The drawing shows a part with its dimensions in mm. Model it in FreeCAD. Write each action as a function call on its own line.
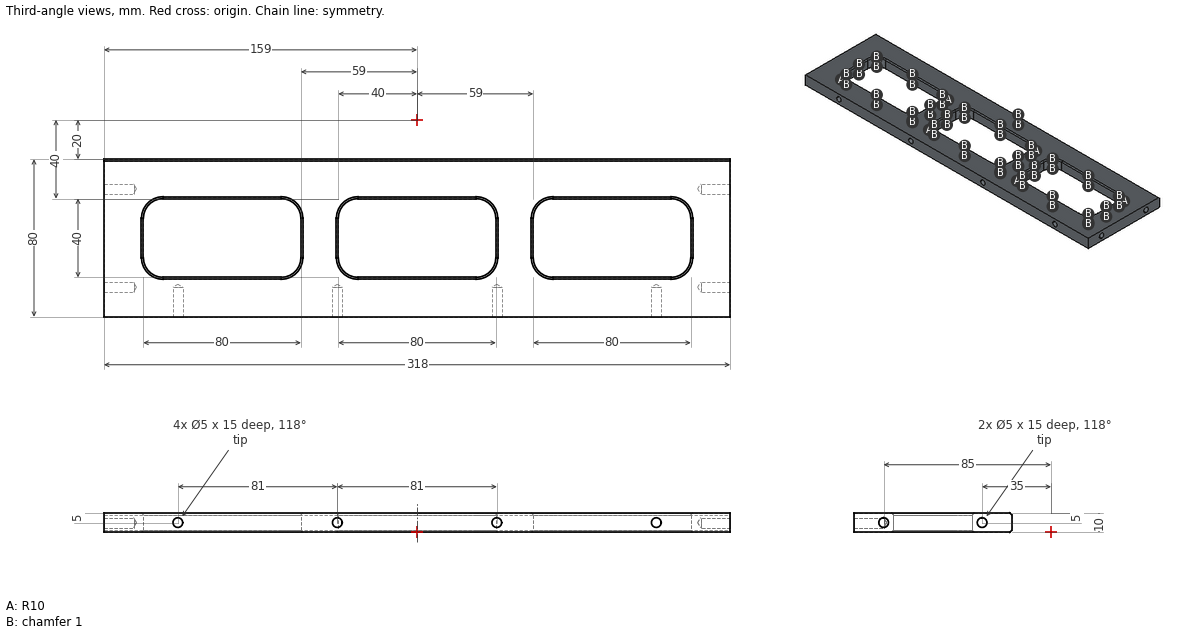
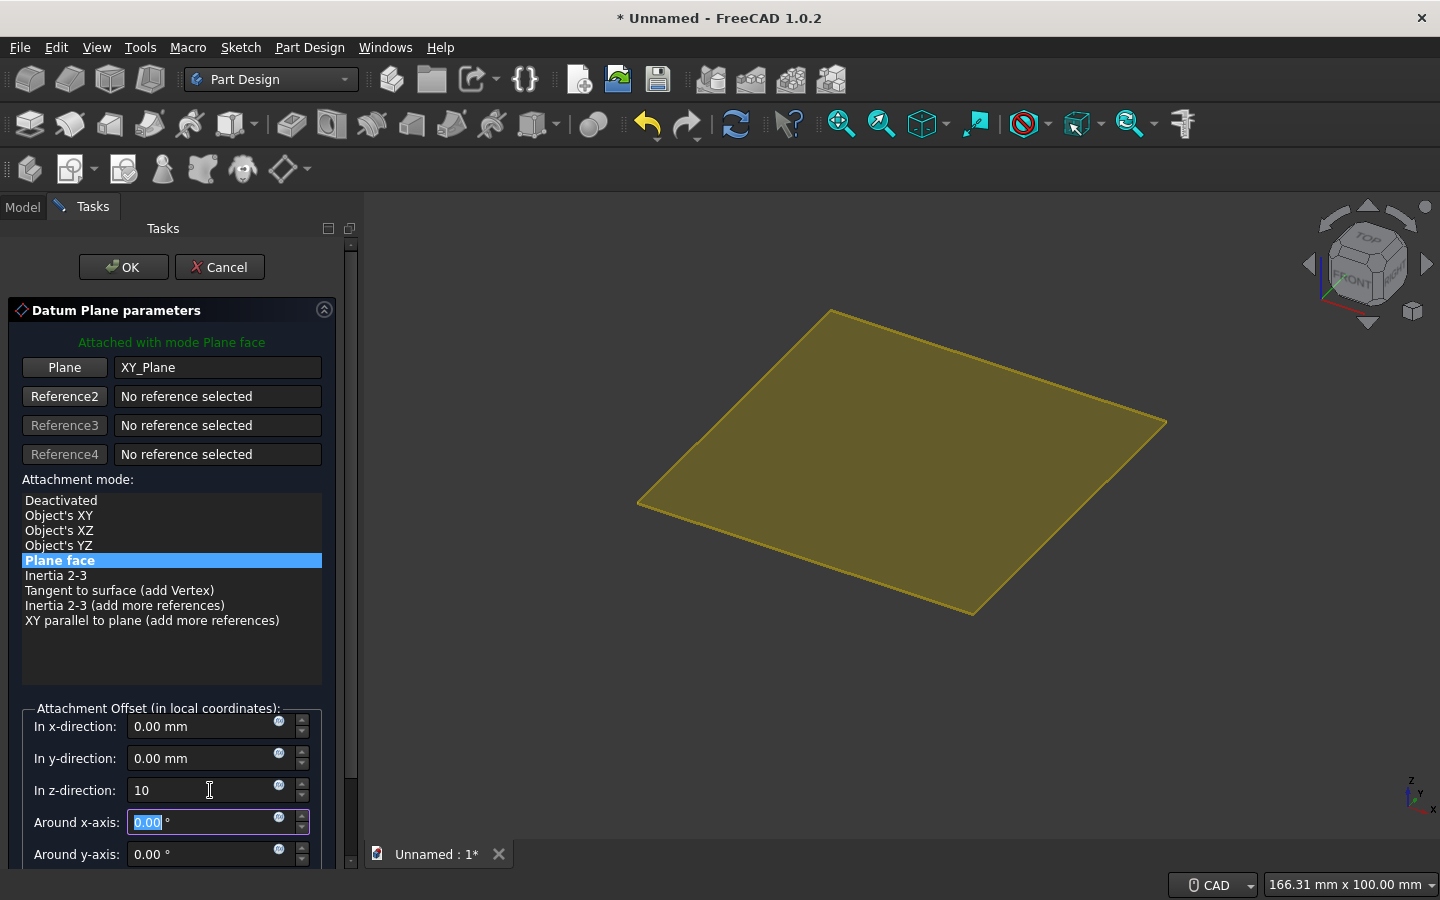
click(124, 267)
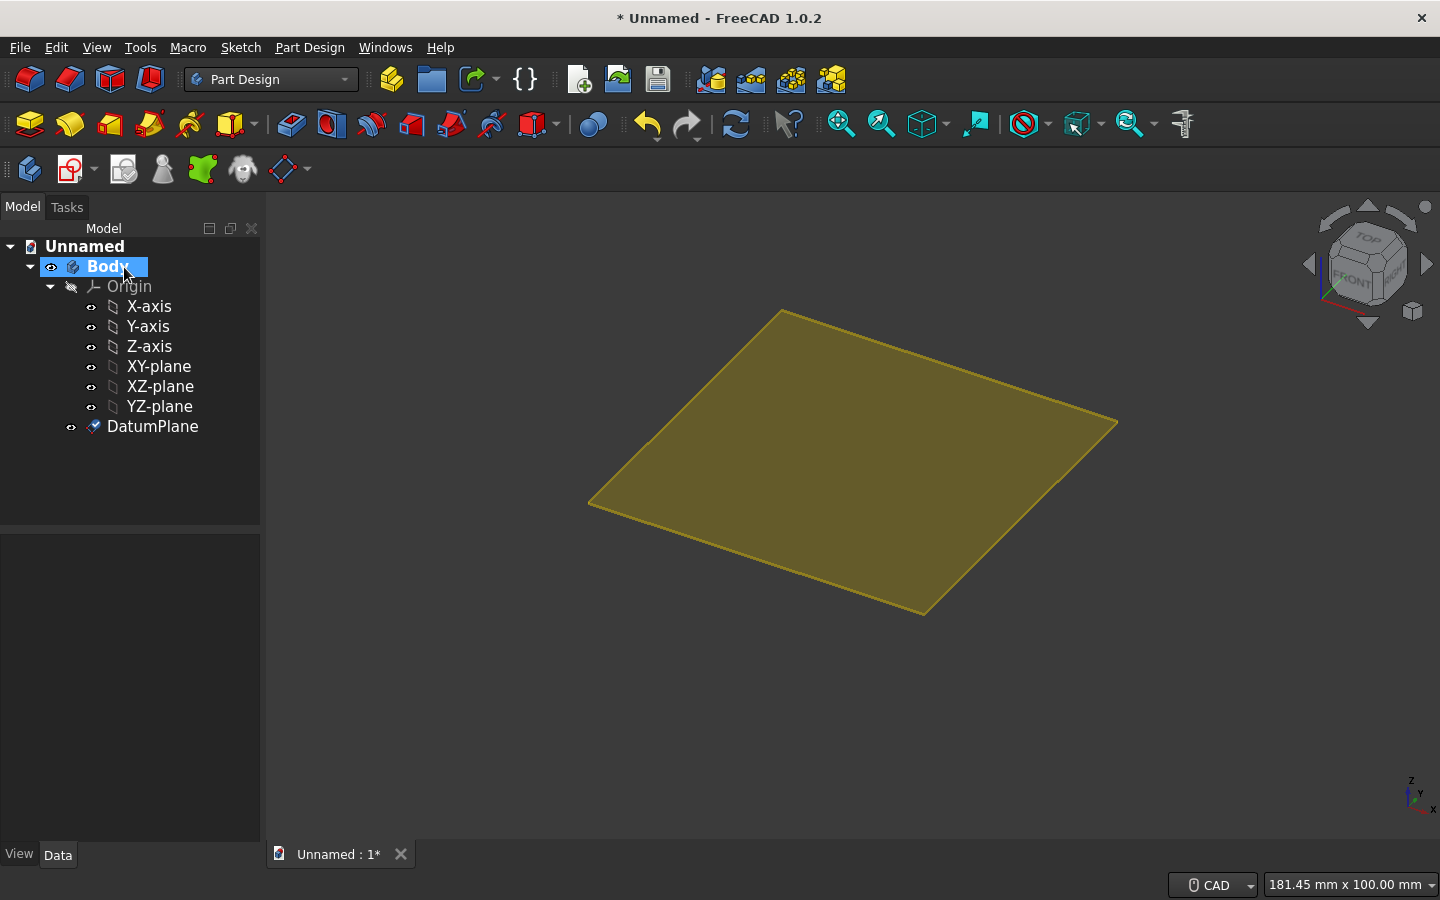
click(116, 427)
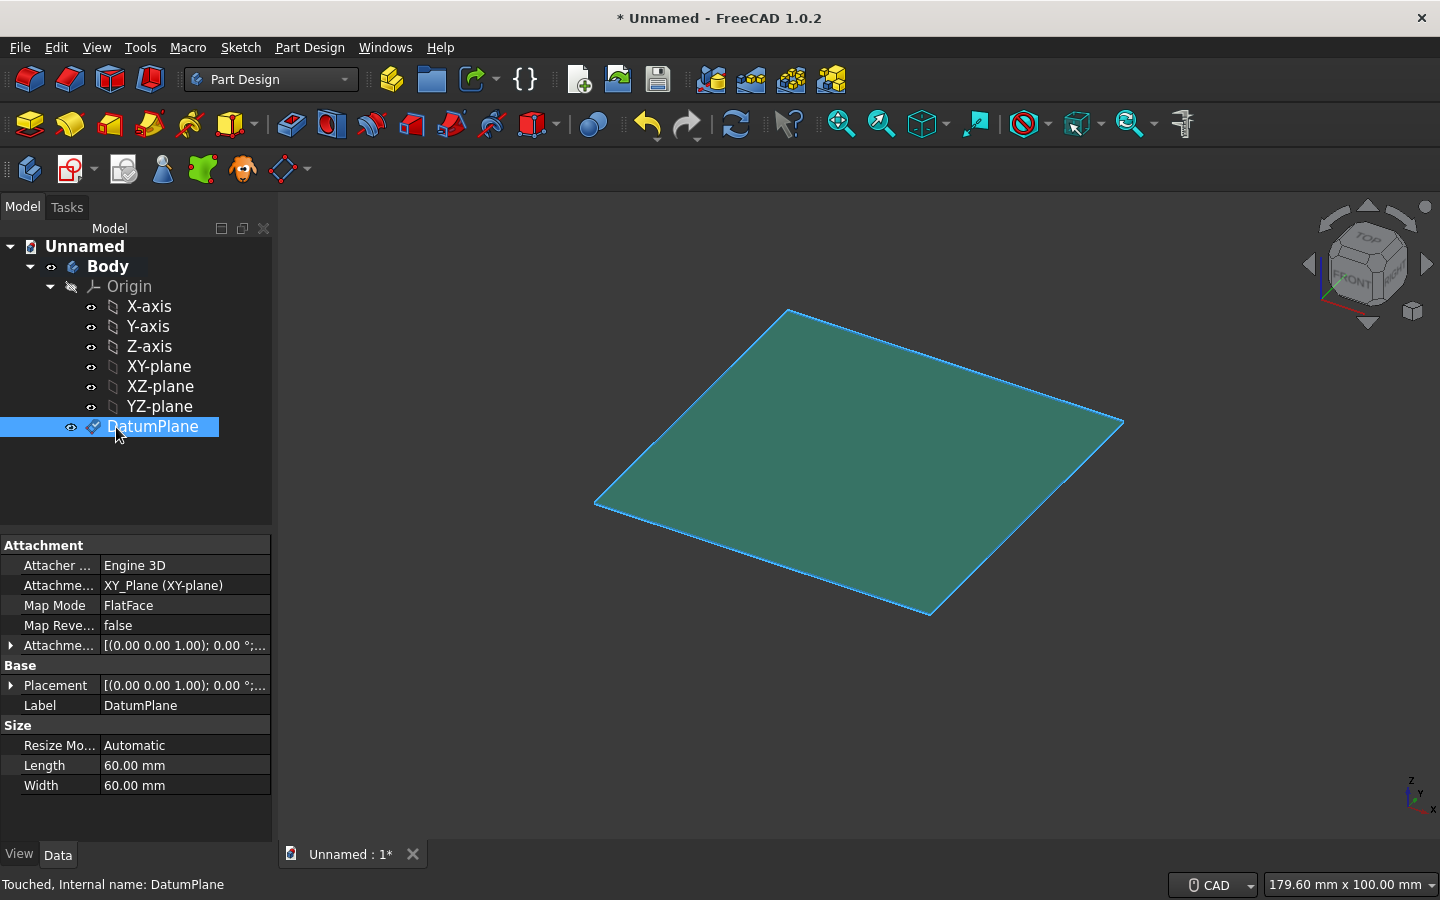
click(70, 170)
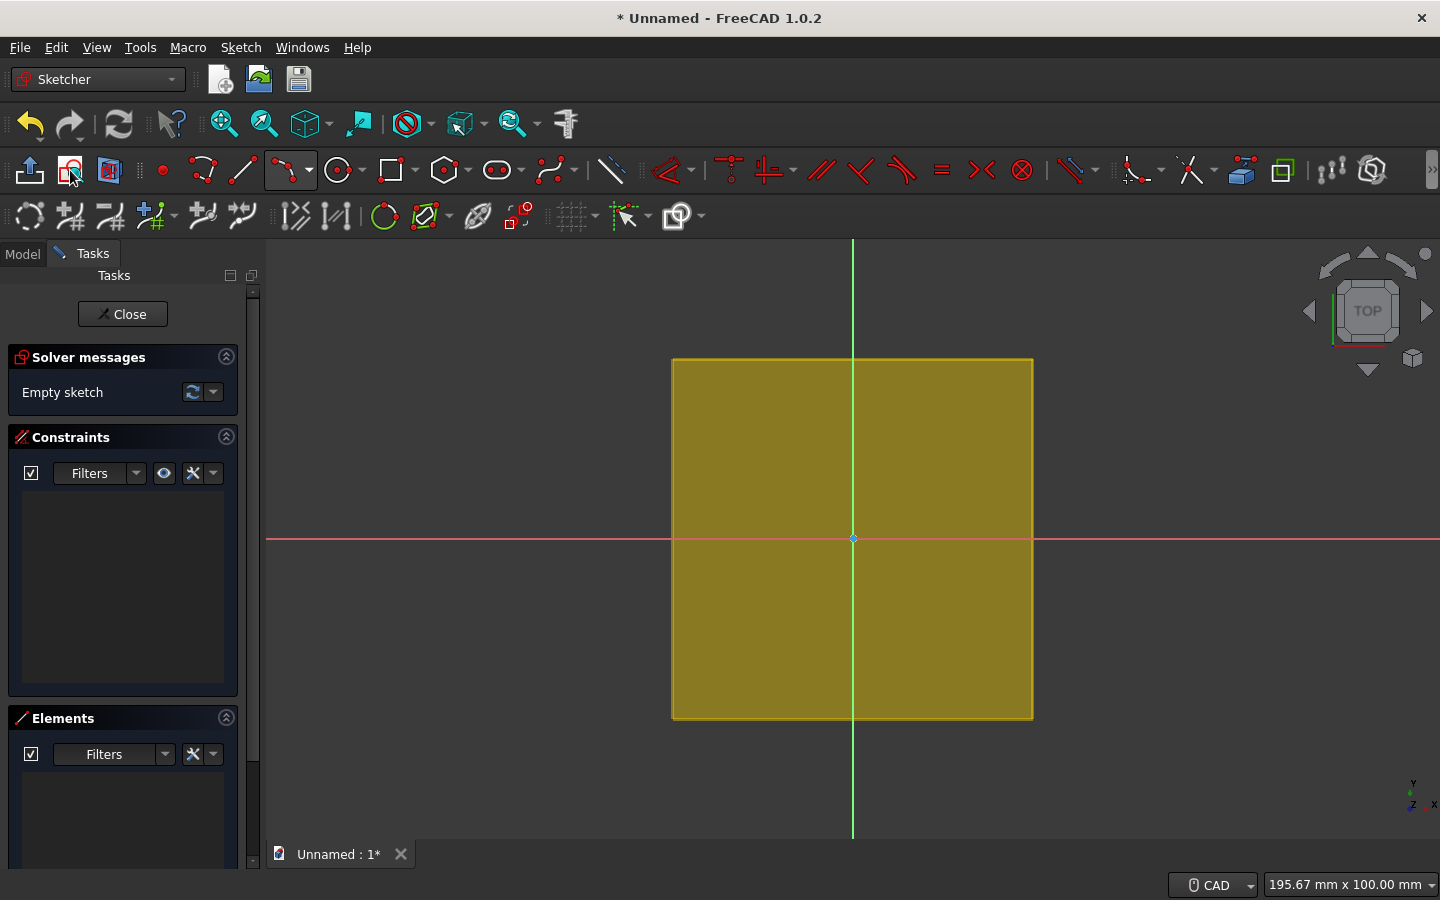
scroll(745, 364, down, 5)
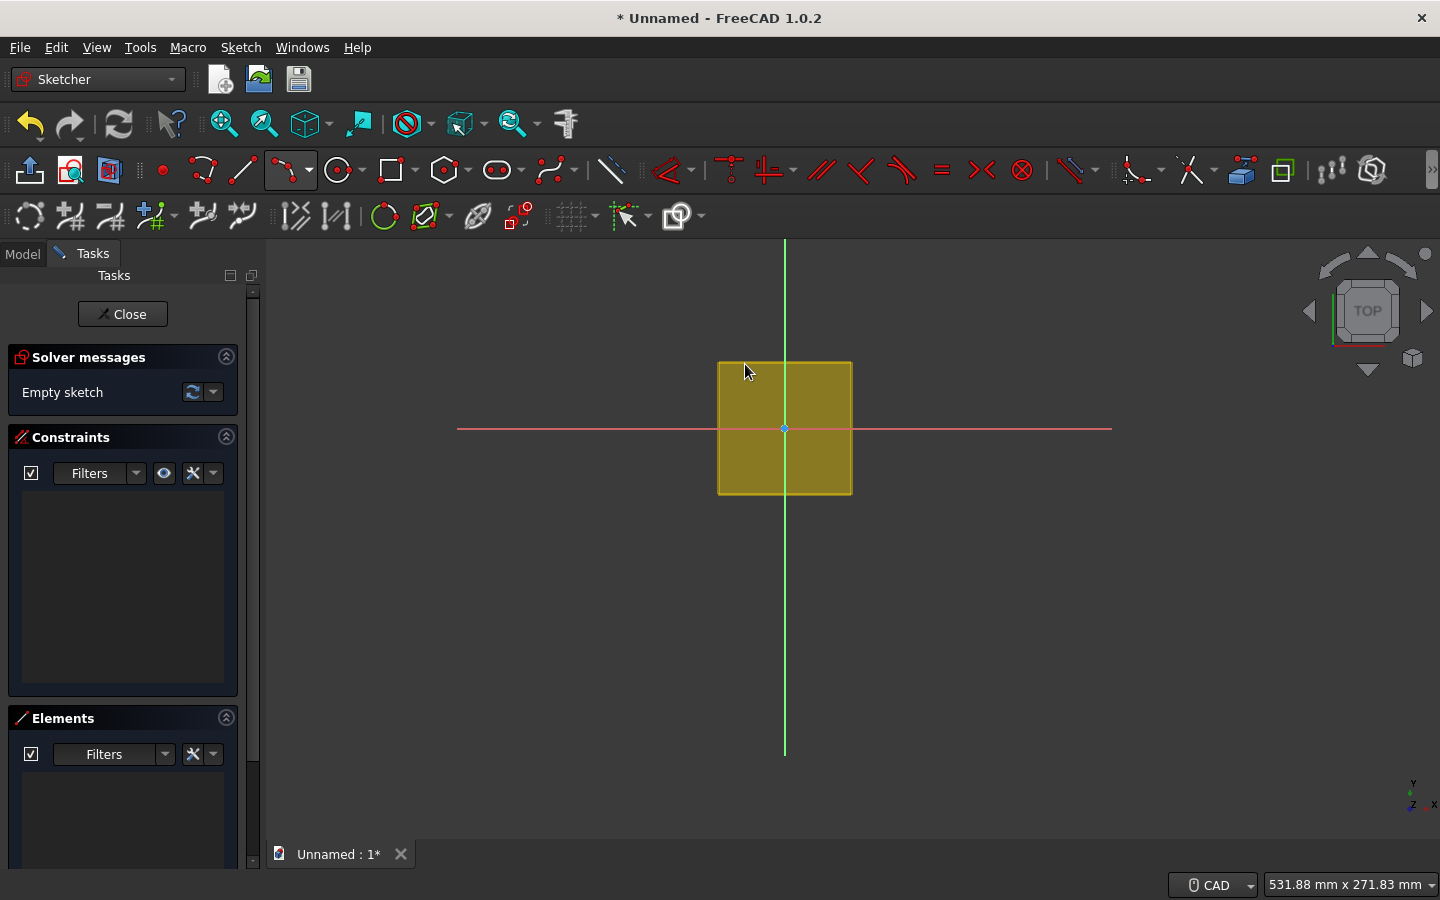
click(392, 170)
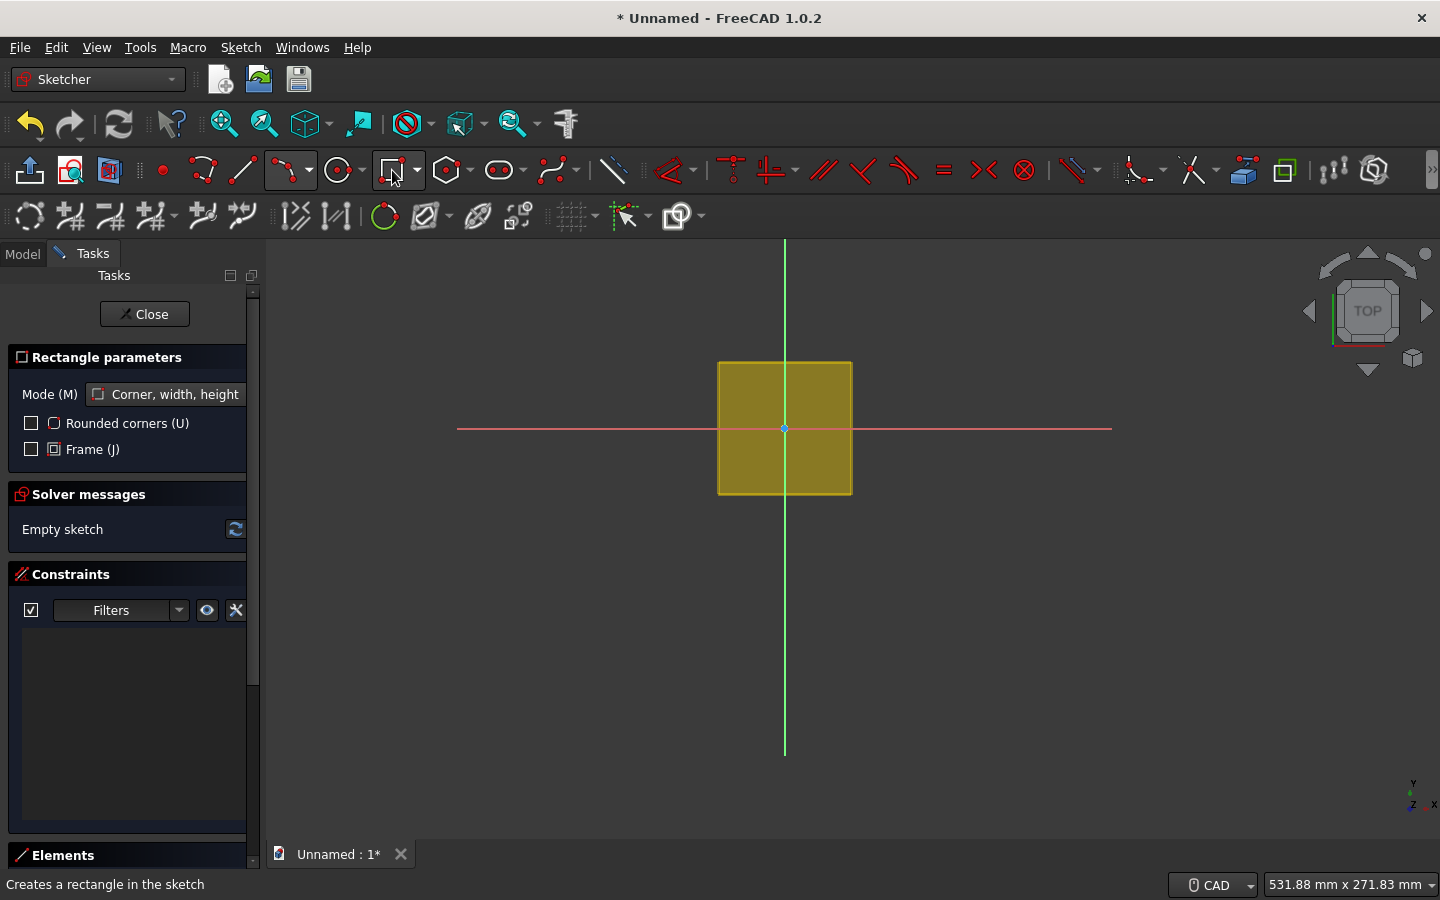
click(434, 473)
click(1136, 649)
key(Escape)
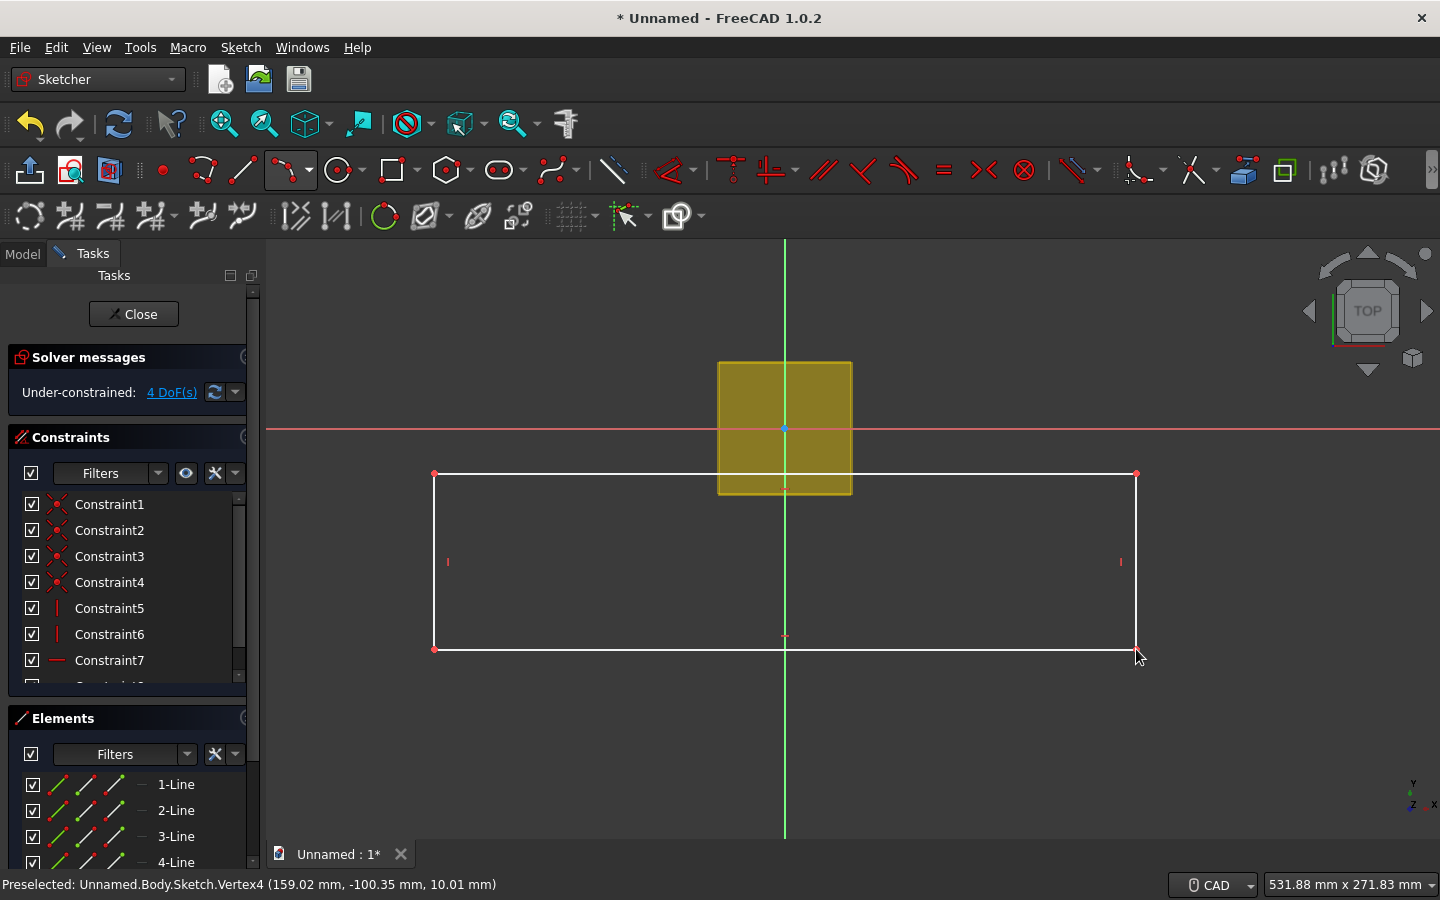
click(668, 170)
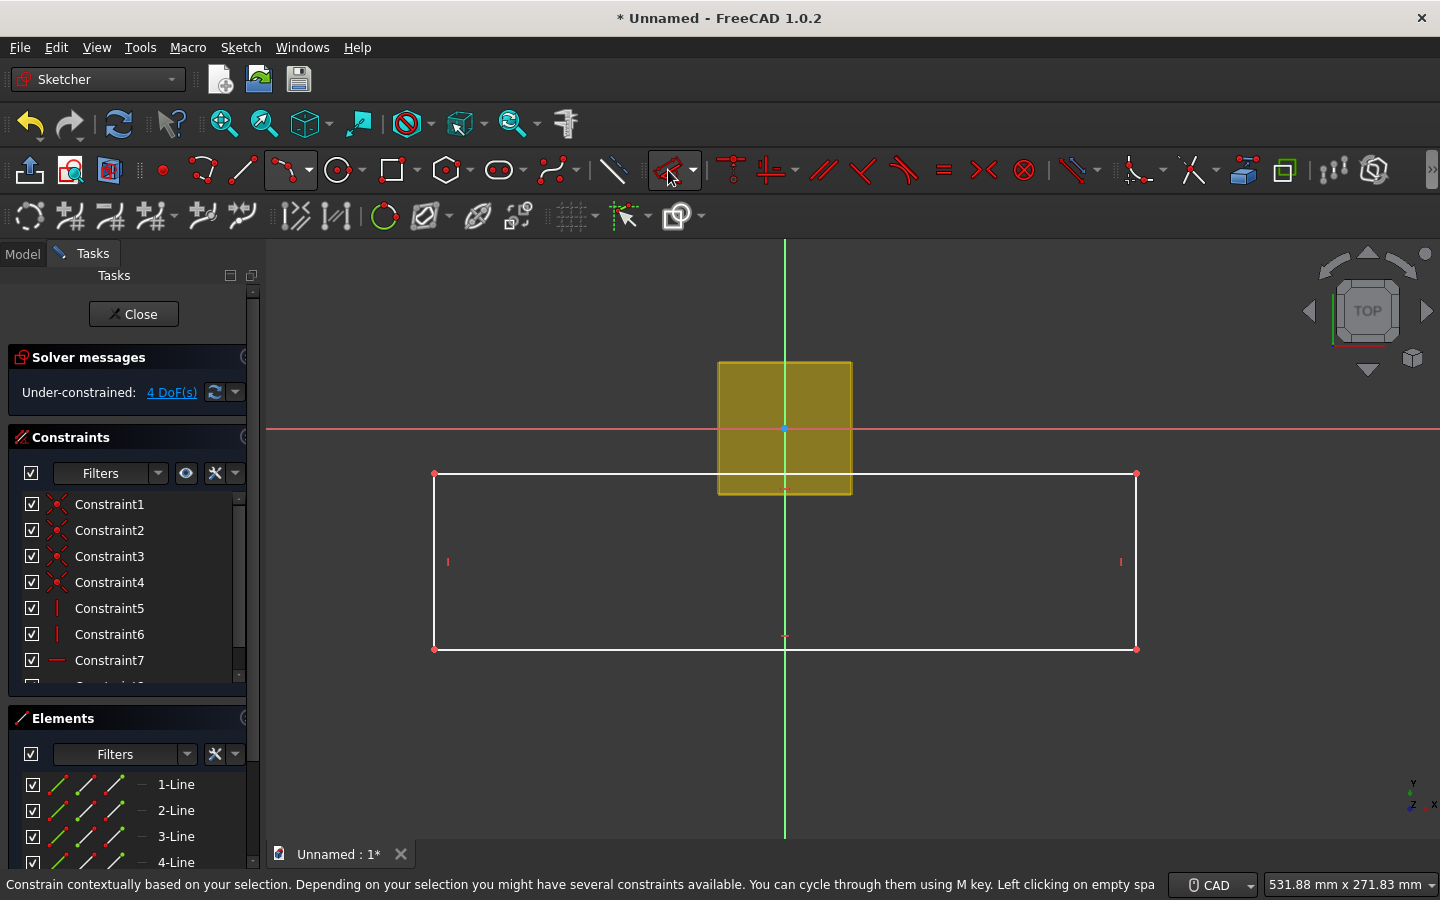
click(434, 527)
click(400, 562)